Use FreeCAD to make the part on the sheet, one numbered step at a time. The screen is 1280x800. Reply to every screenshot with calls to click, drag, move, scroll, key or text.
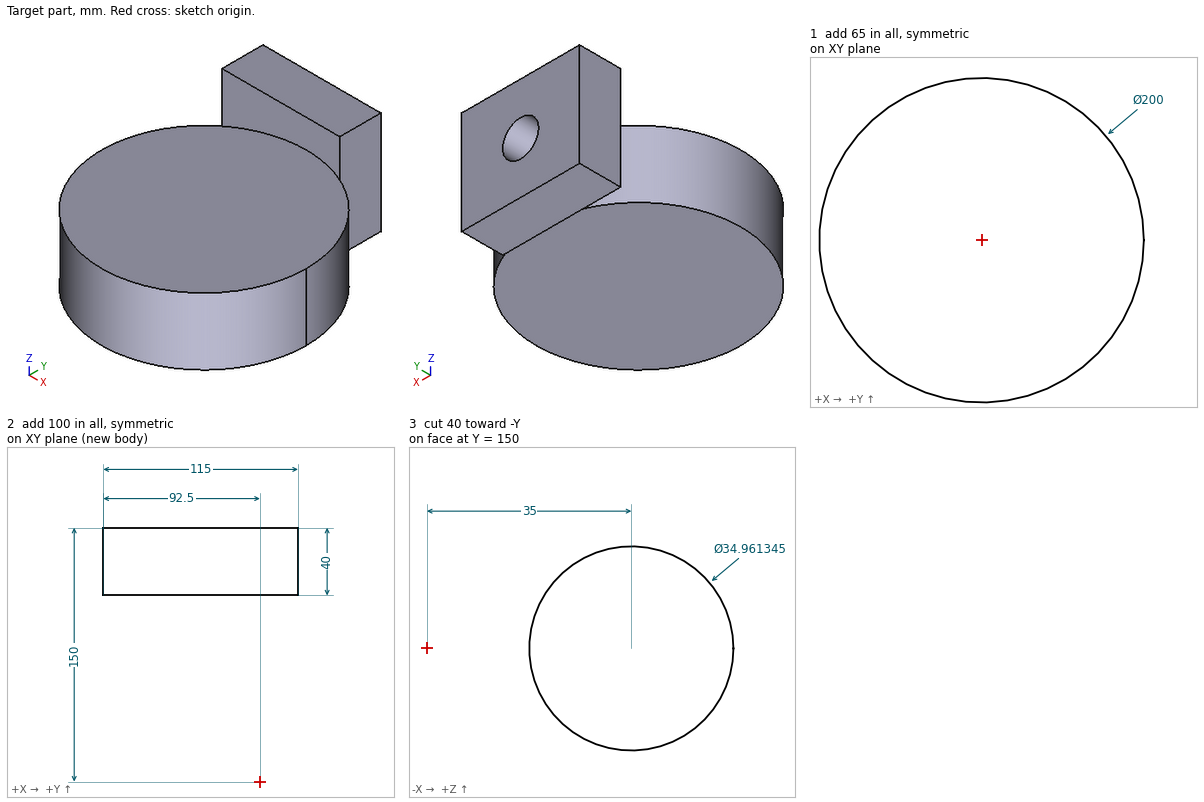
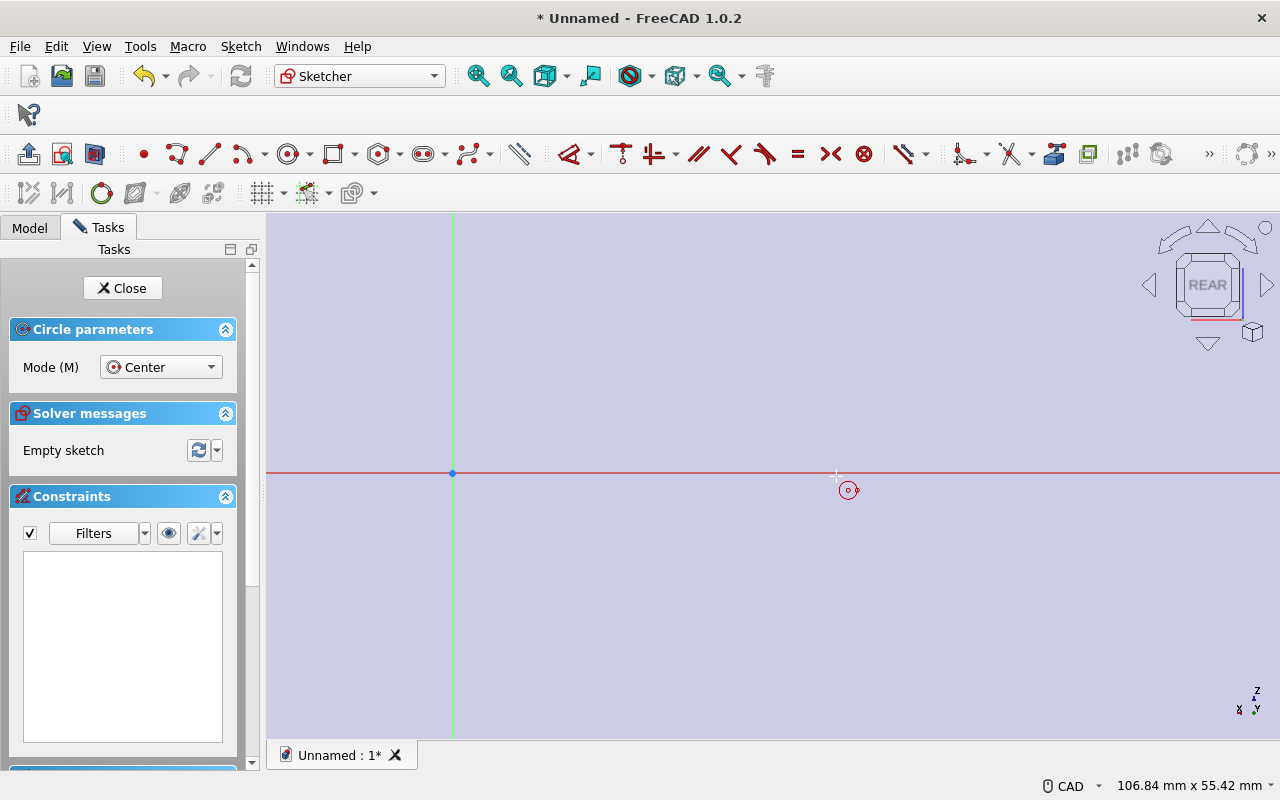
click(785, 473)
move(902, 356)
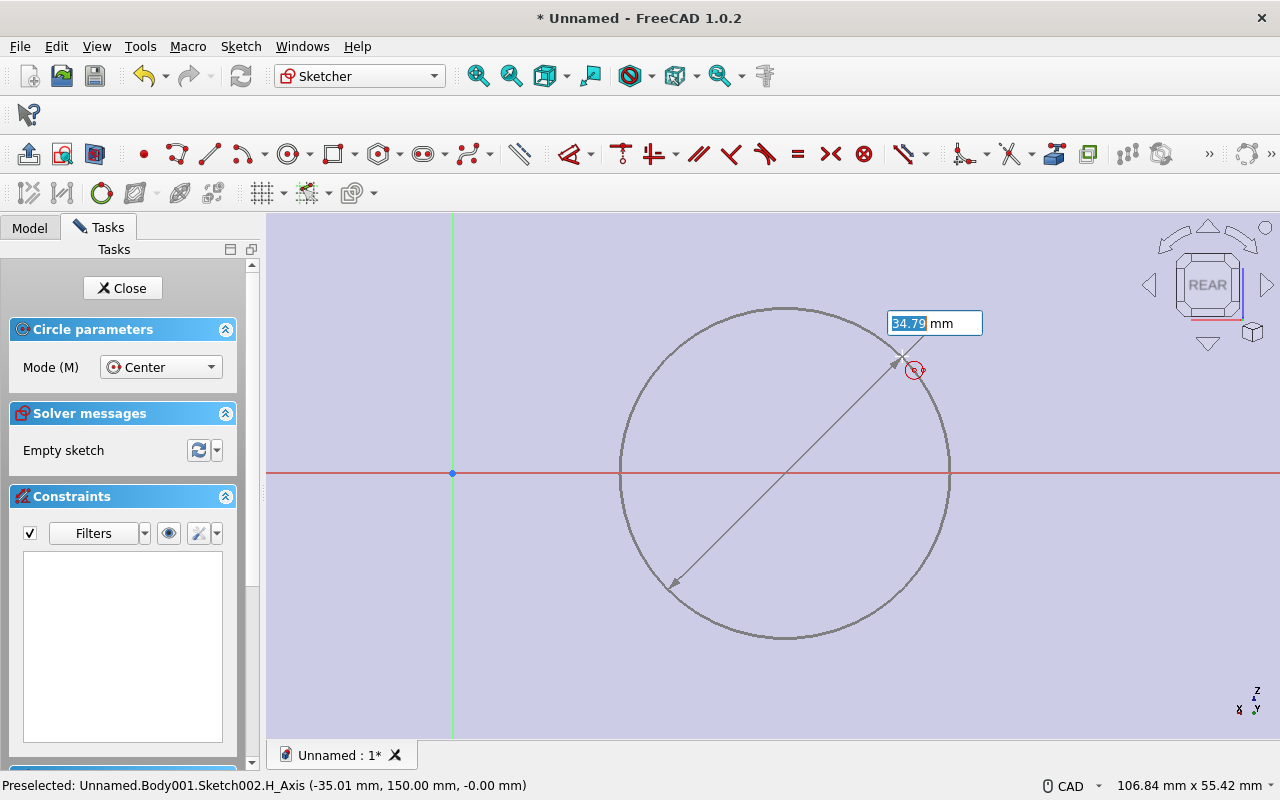
text(34.961345)
key(Return)
key(Escape)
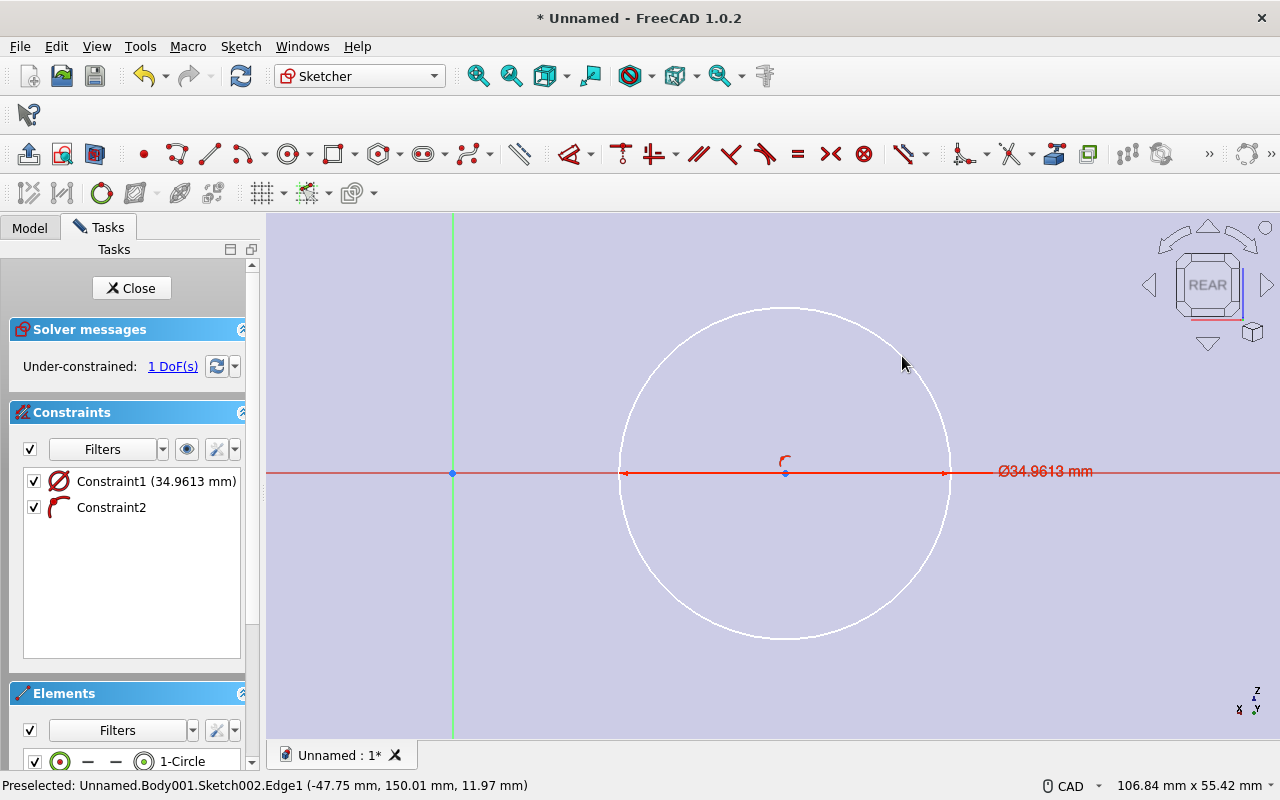
key(d)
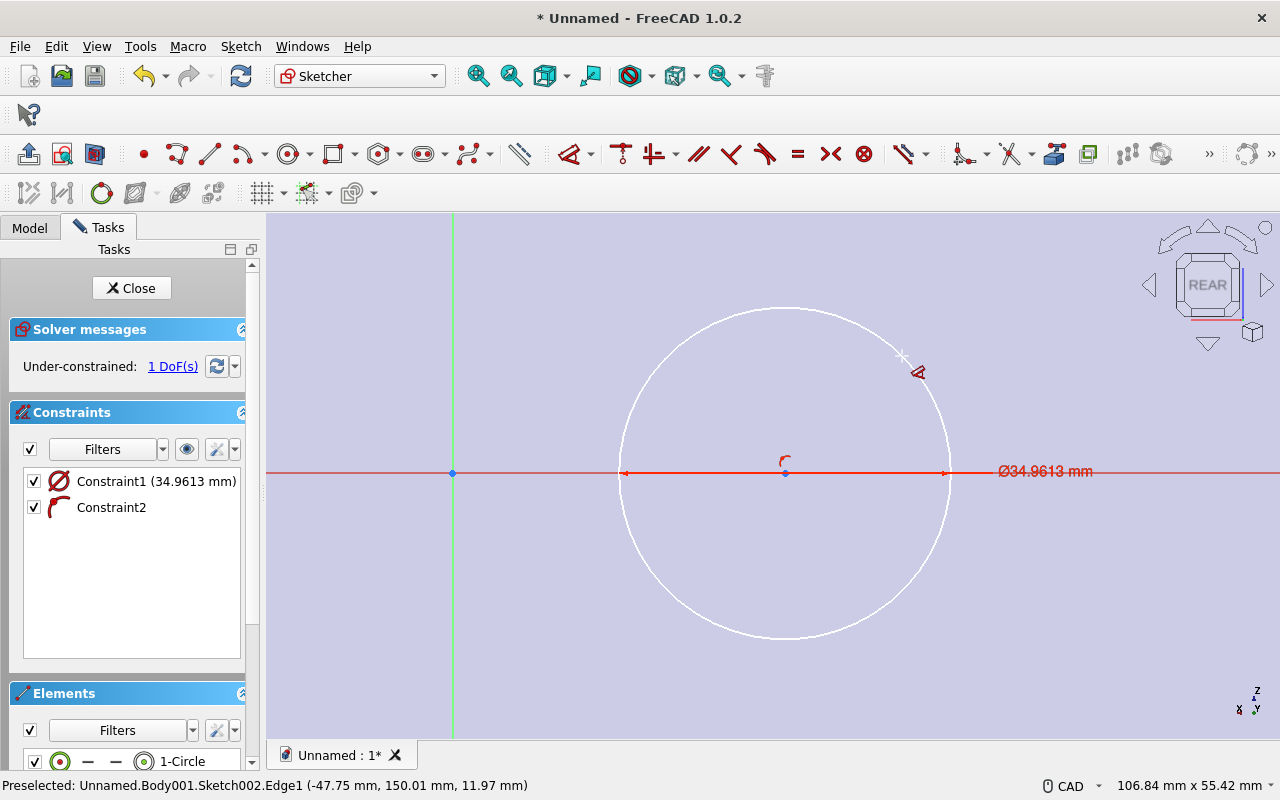
click(785, 473)
click(542, 507)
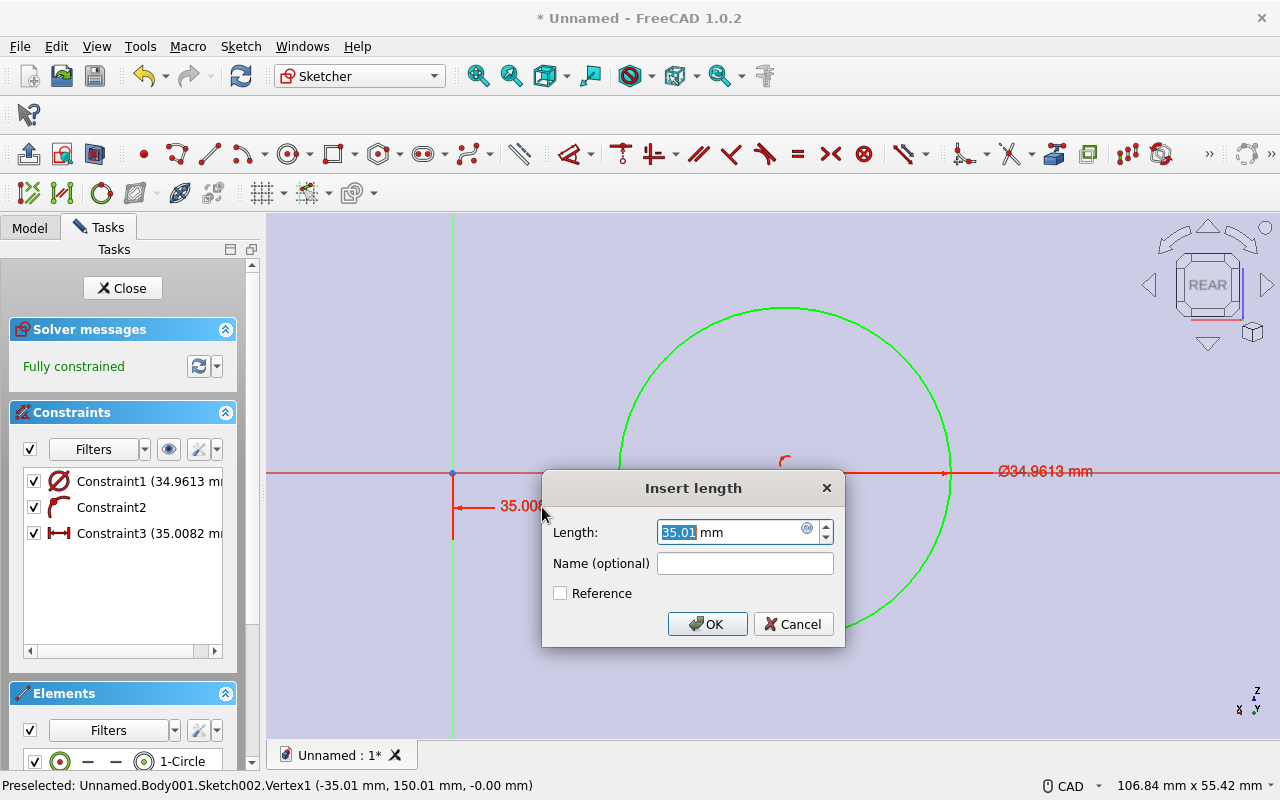
text(35)
key(Return)
key(Escape)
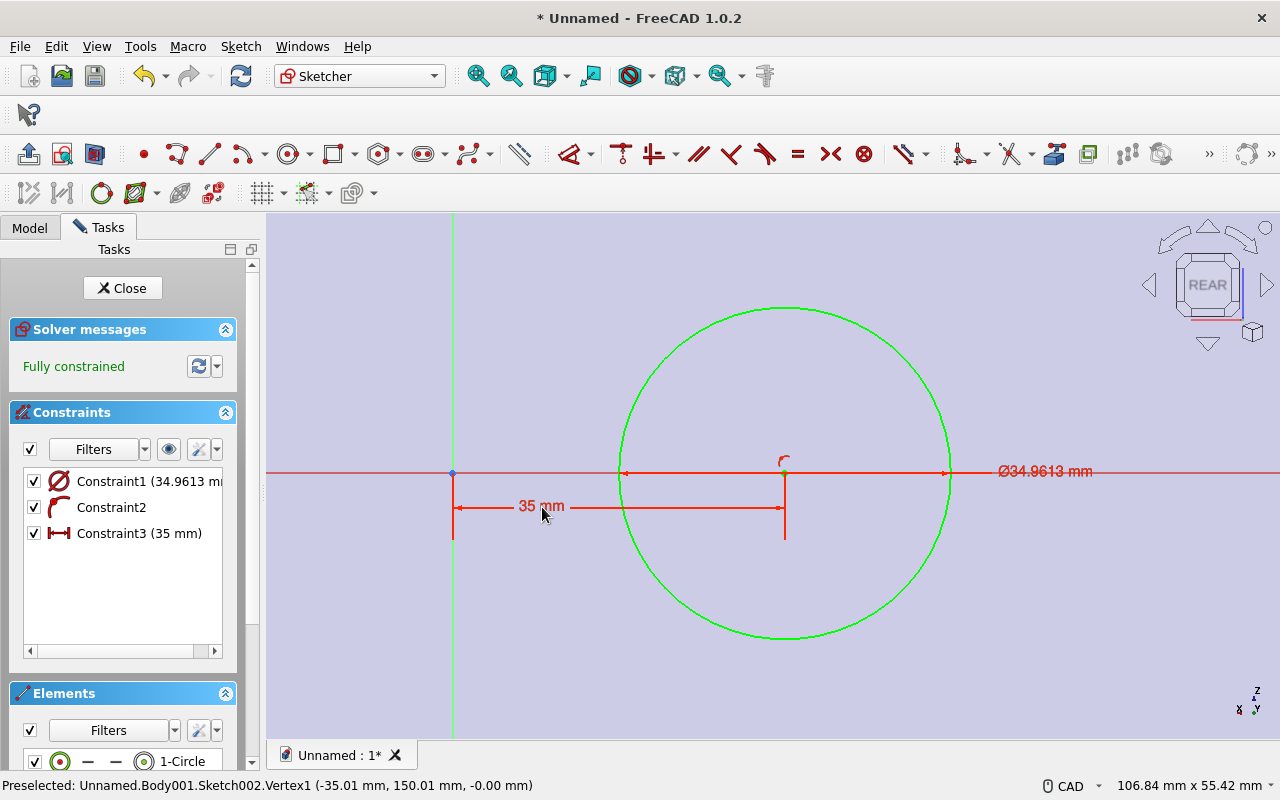
click(123, 288)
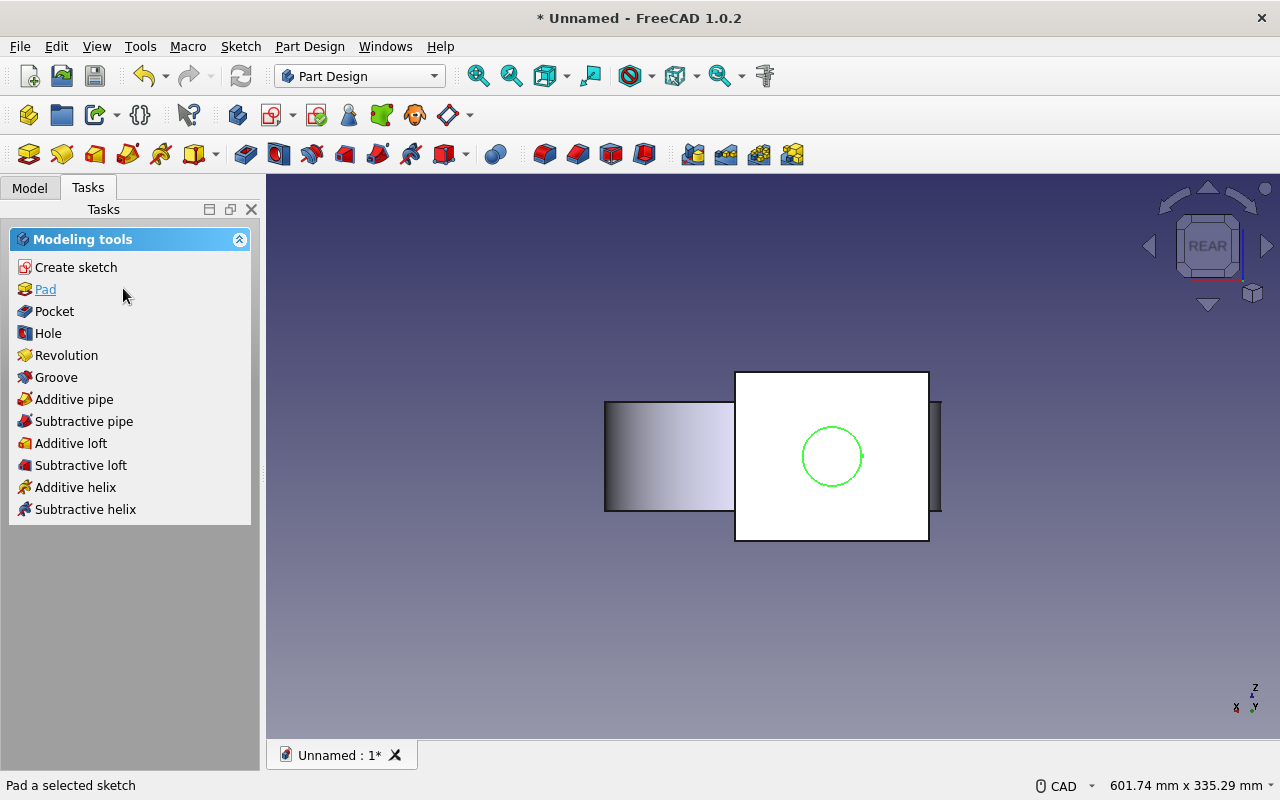
click(246, 154)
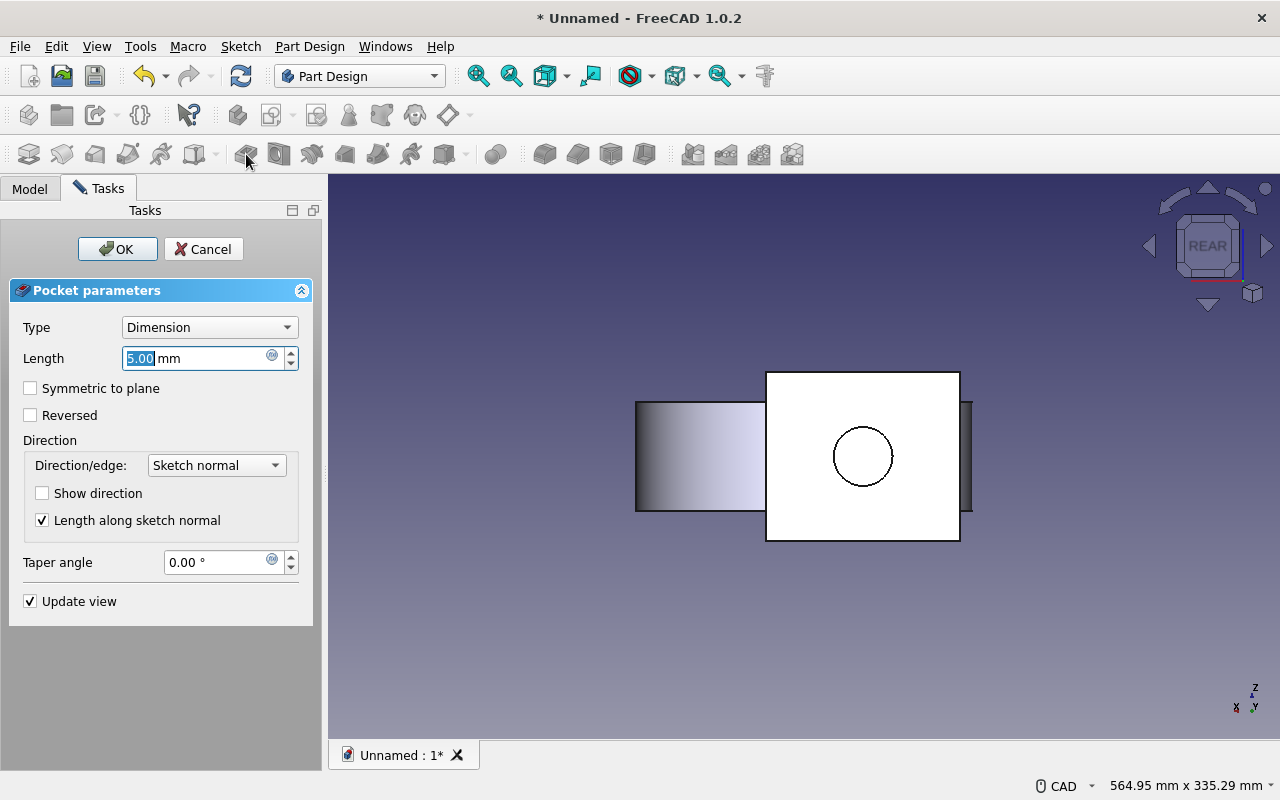
text(40)
key(Tab)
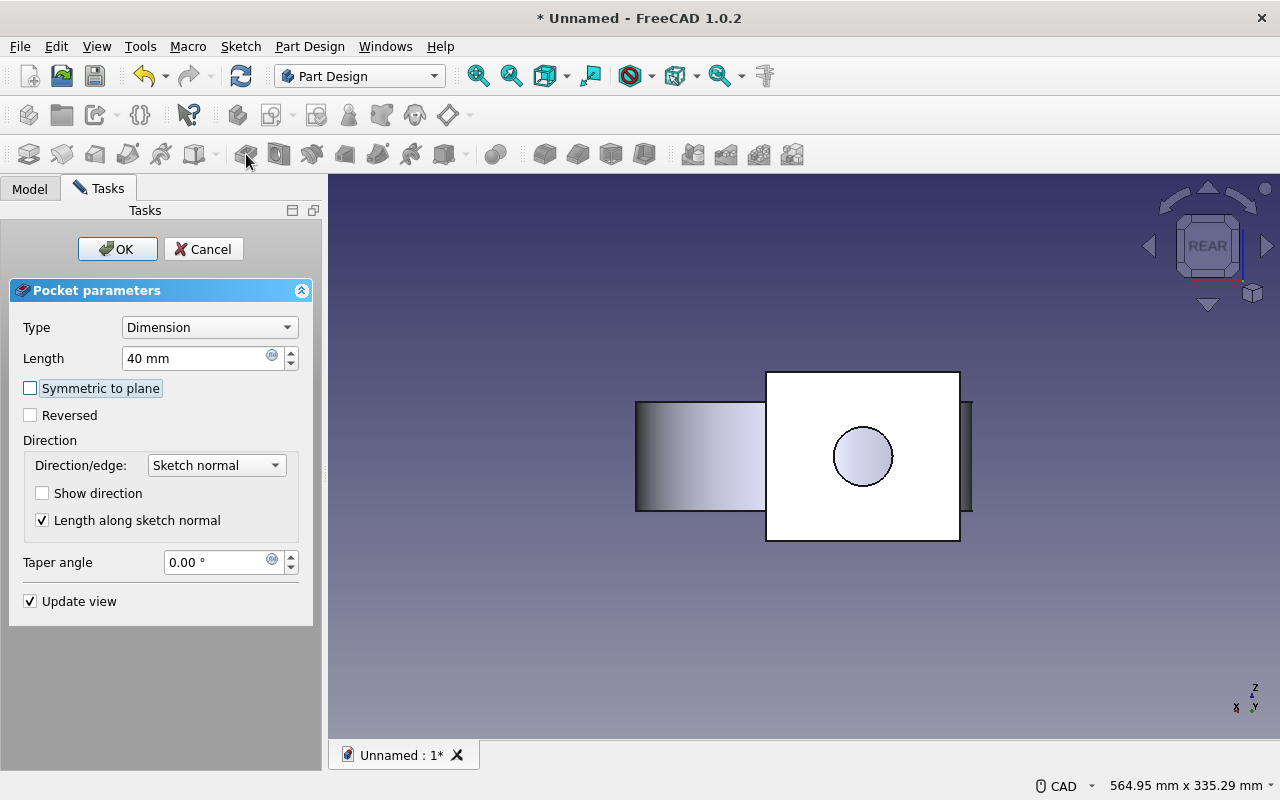
click(118, 249)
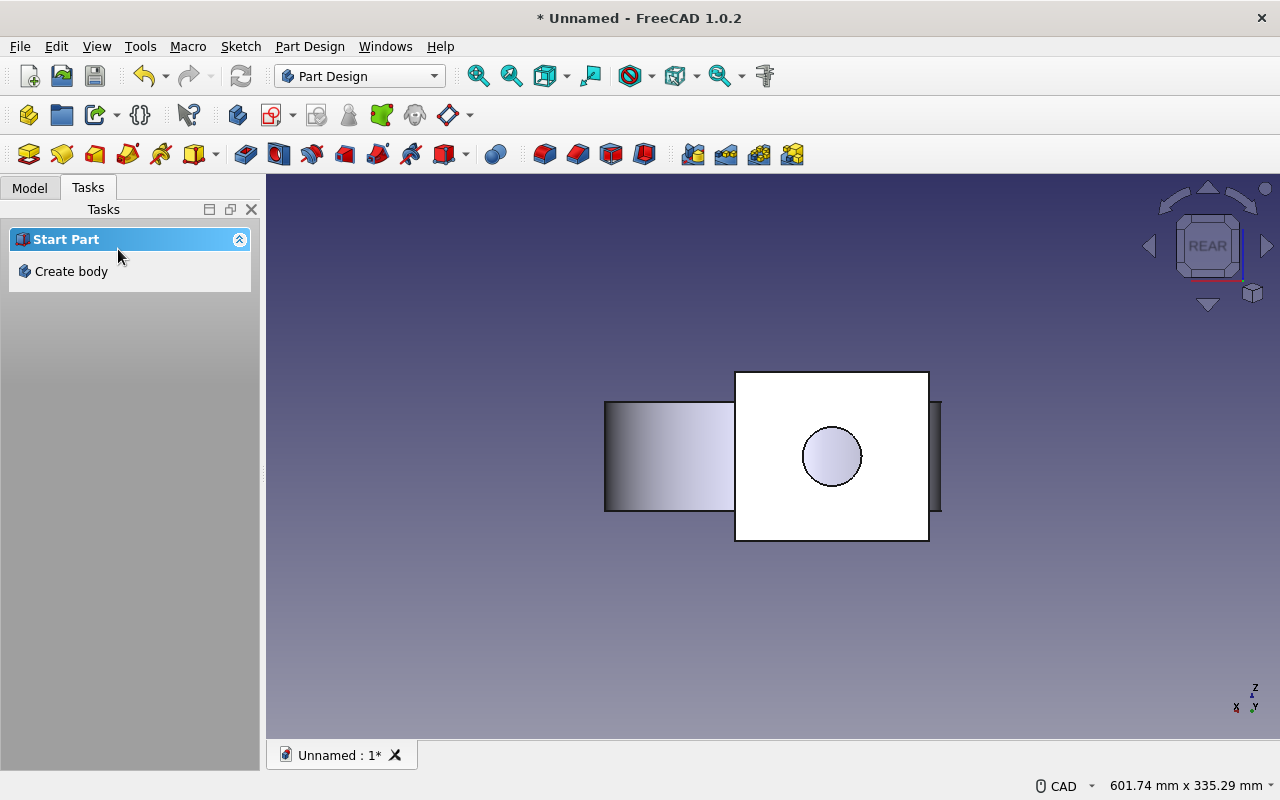
key(0)